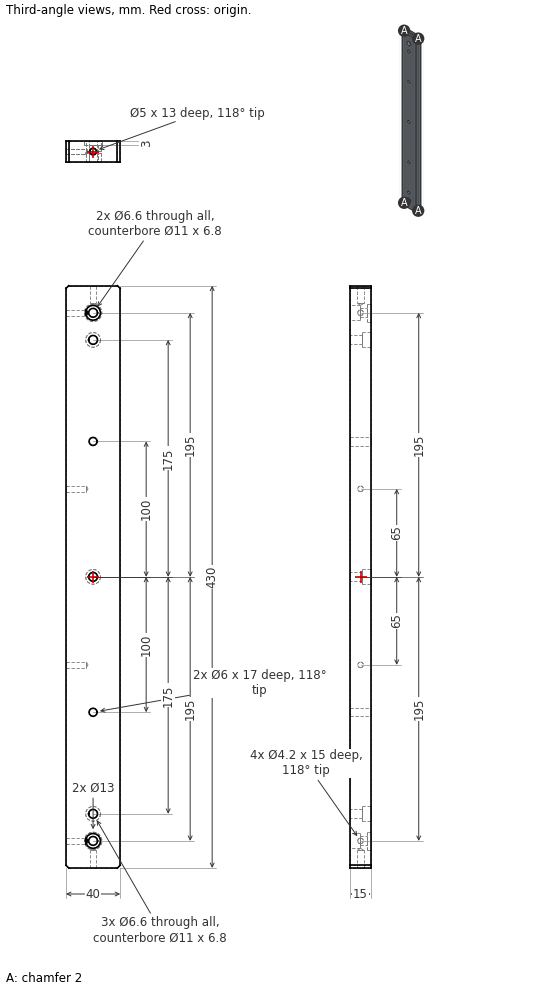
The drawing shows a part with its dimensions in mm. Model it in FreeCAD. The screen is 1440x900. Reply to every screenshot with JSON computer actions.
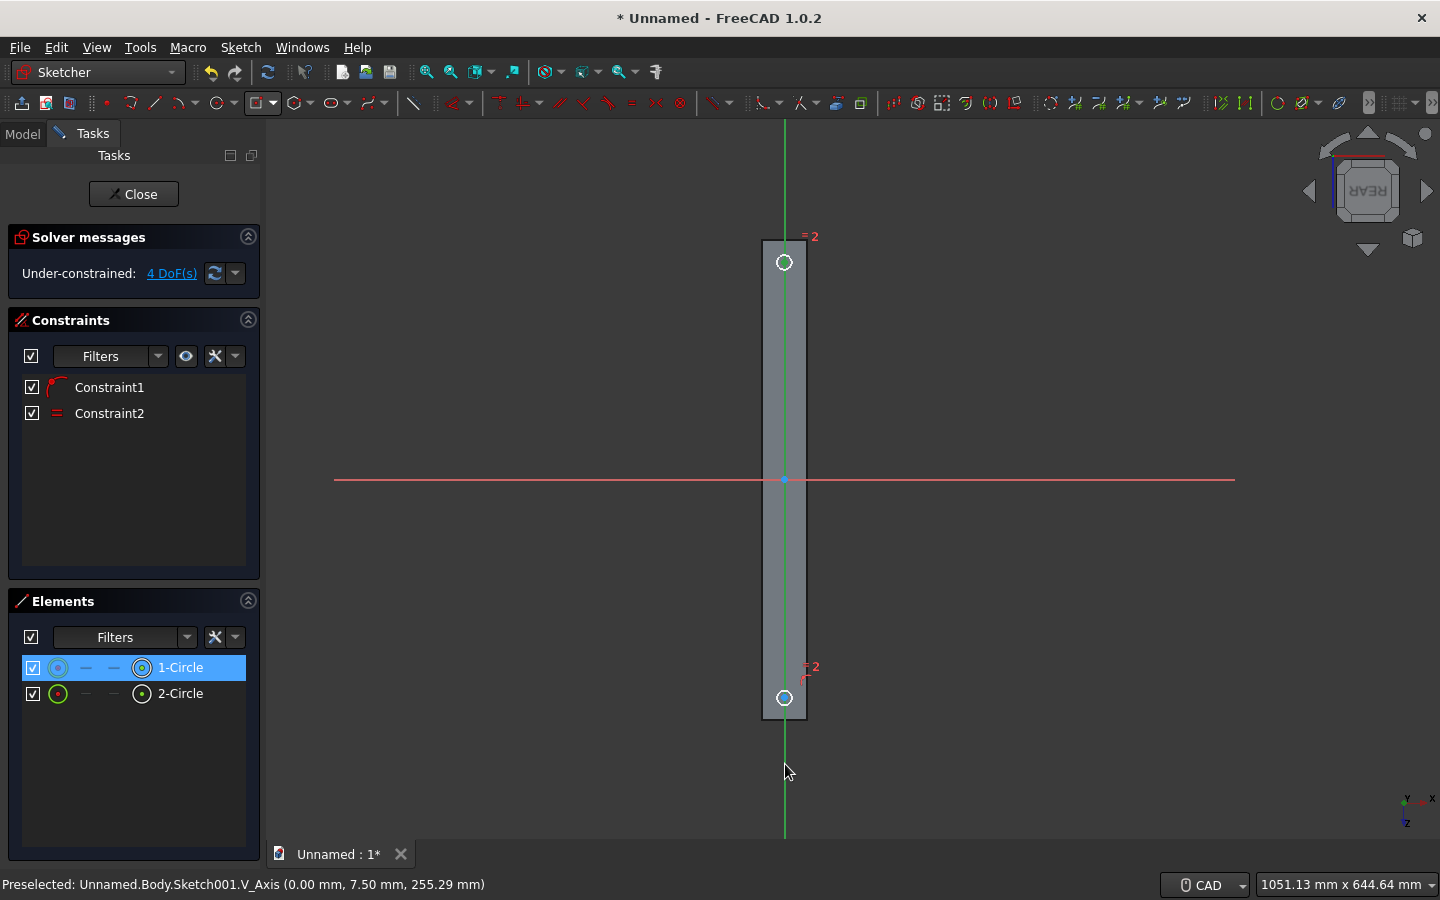
{"action": "left_click", "coordinate": [500, 104]}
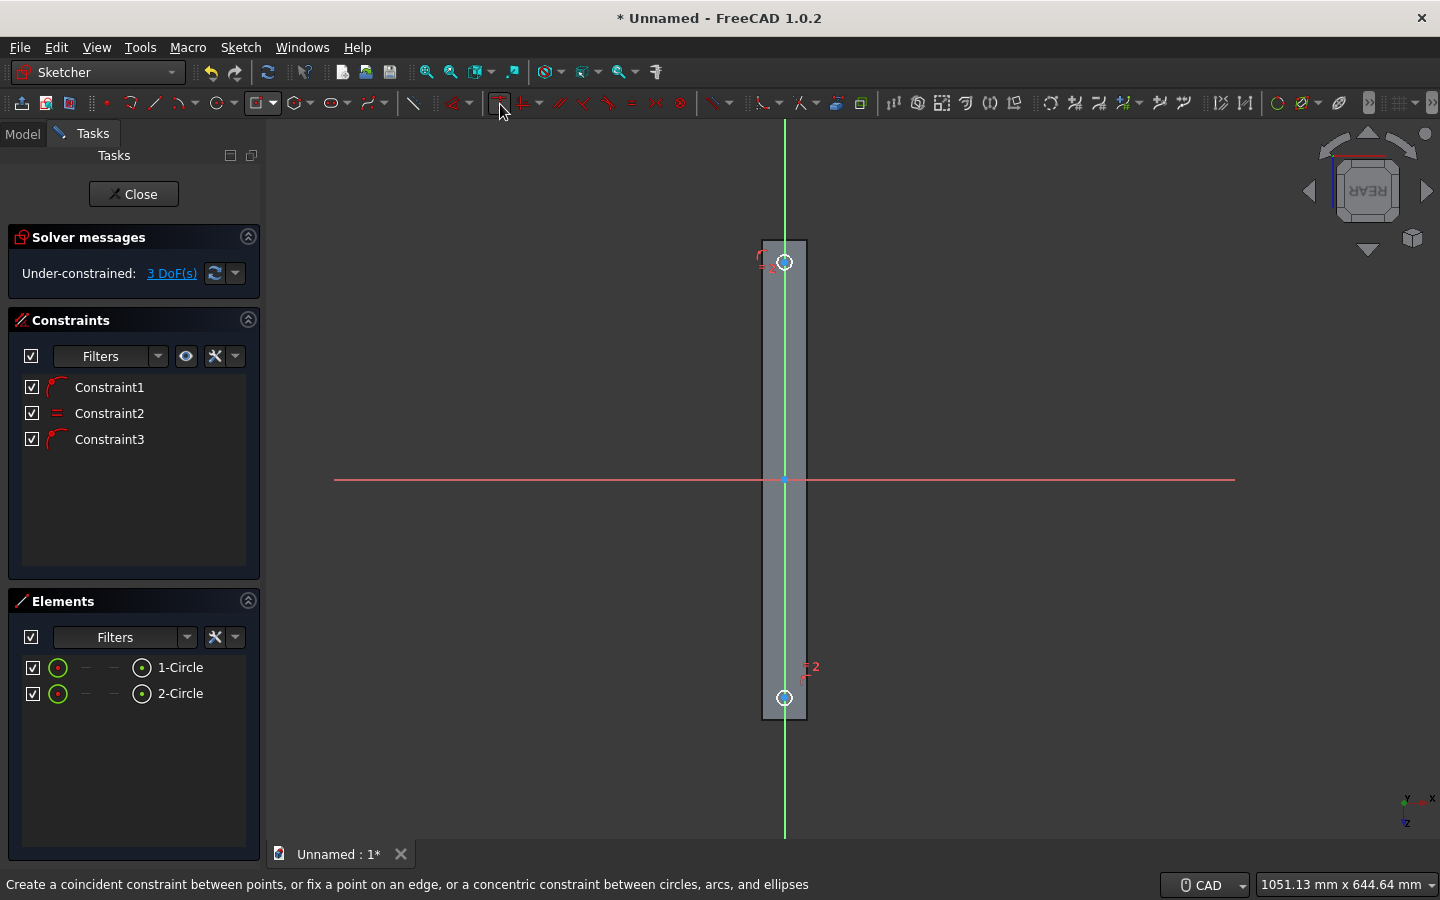
{"action": "key", "text": "d"}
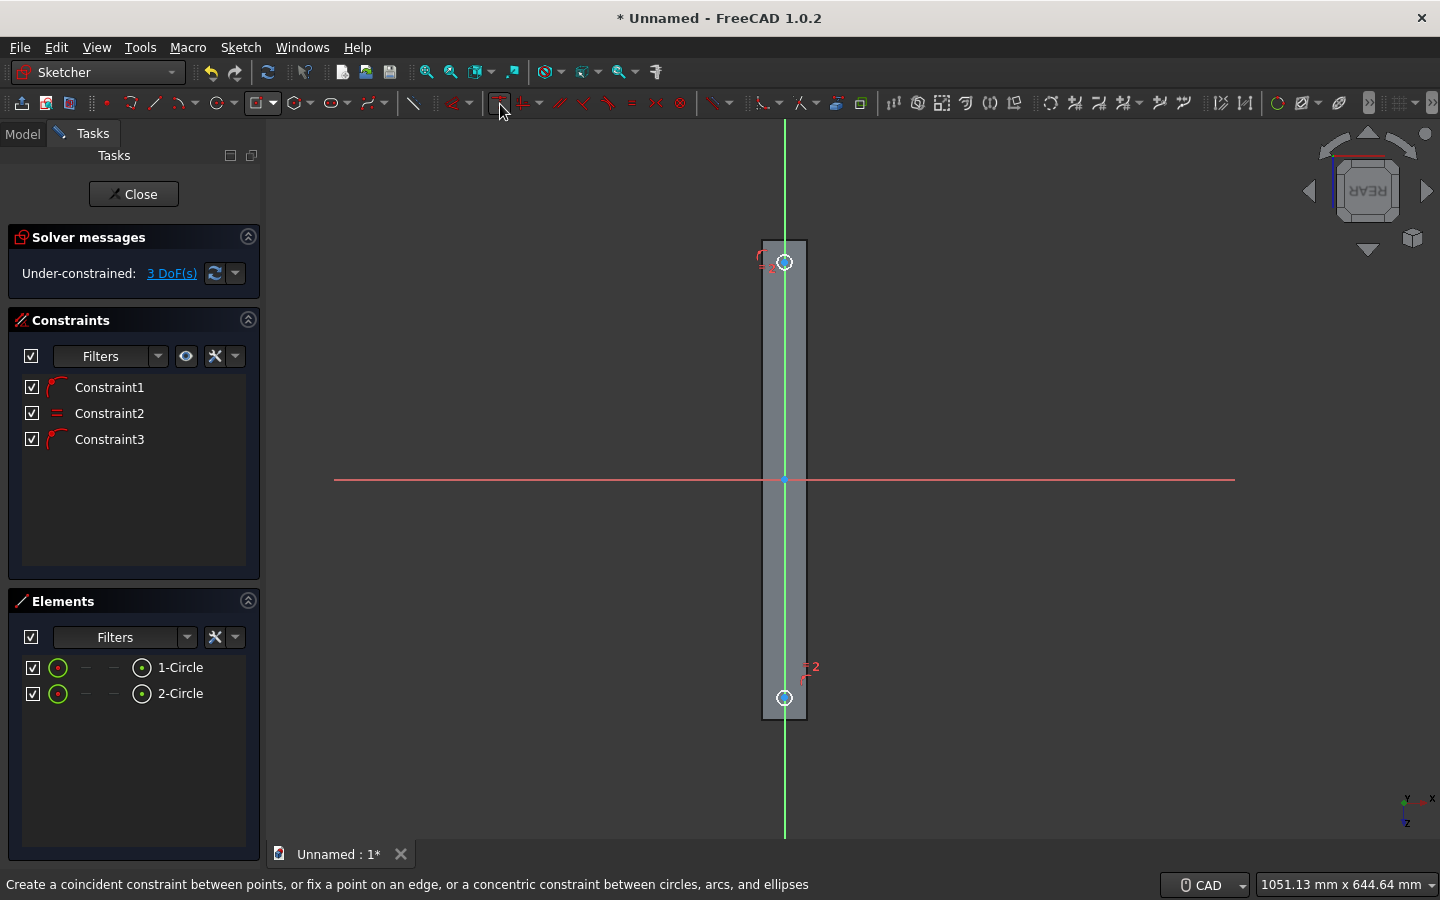
{"action": "scroll", "coordinate": [785, 255], "scroll_direction": "up", "scroll_amount": 6}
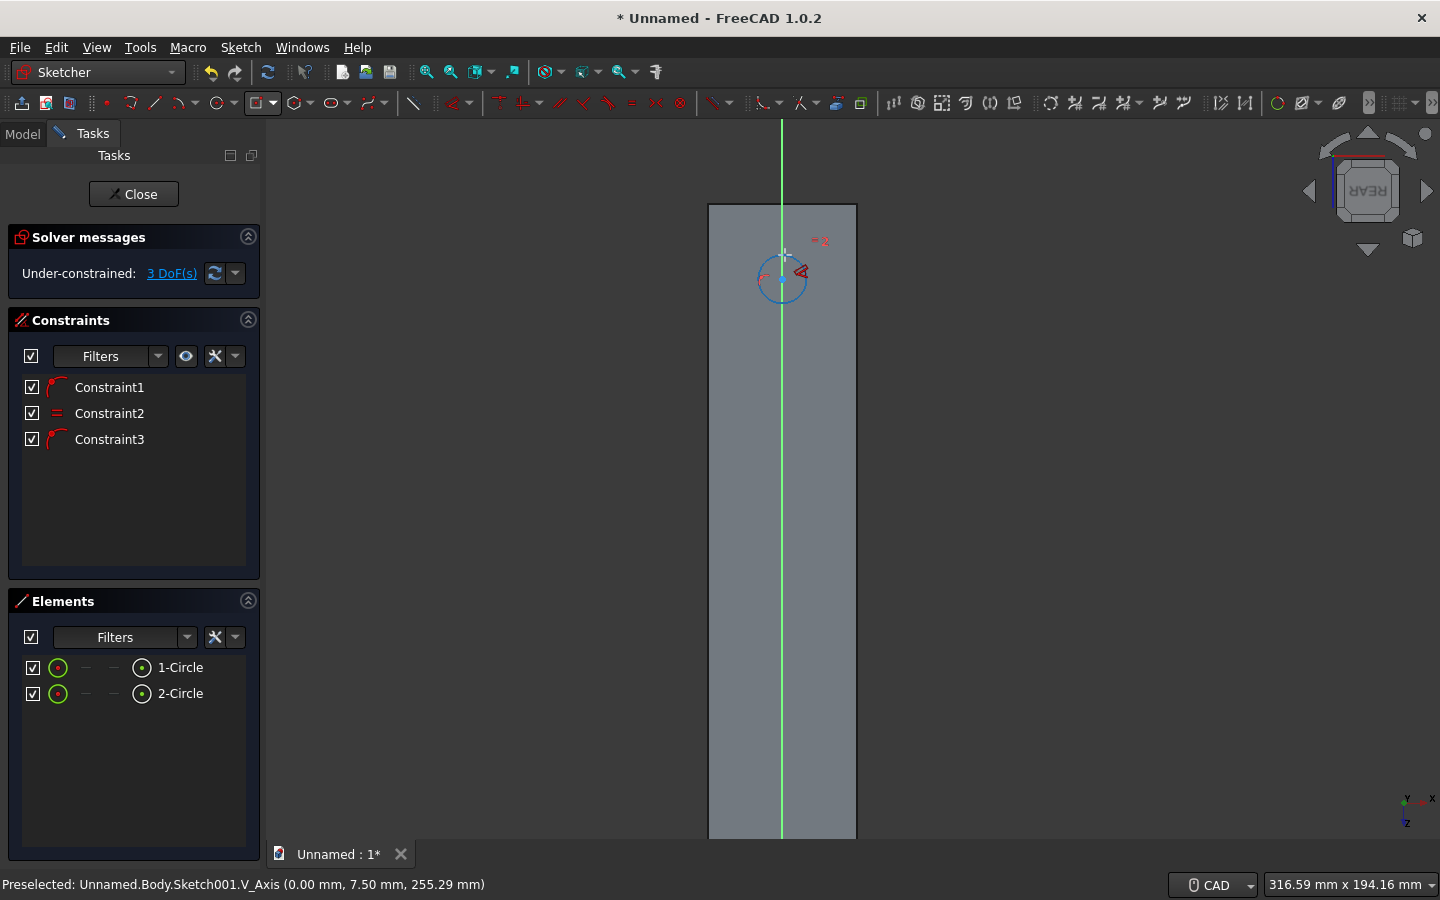
{"action": "left_click", "coordinate": [783, 255]}
{"action": "left_click", "coordinate": [811, 231]}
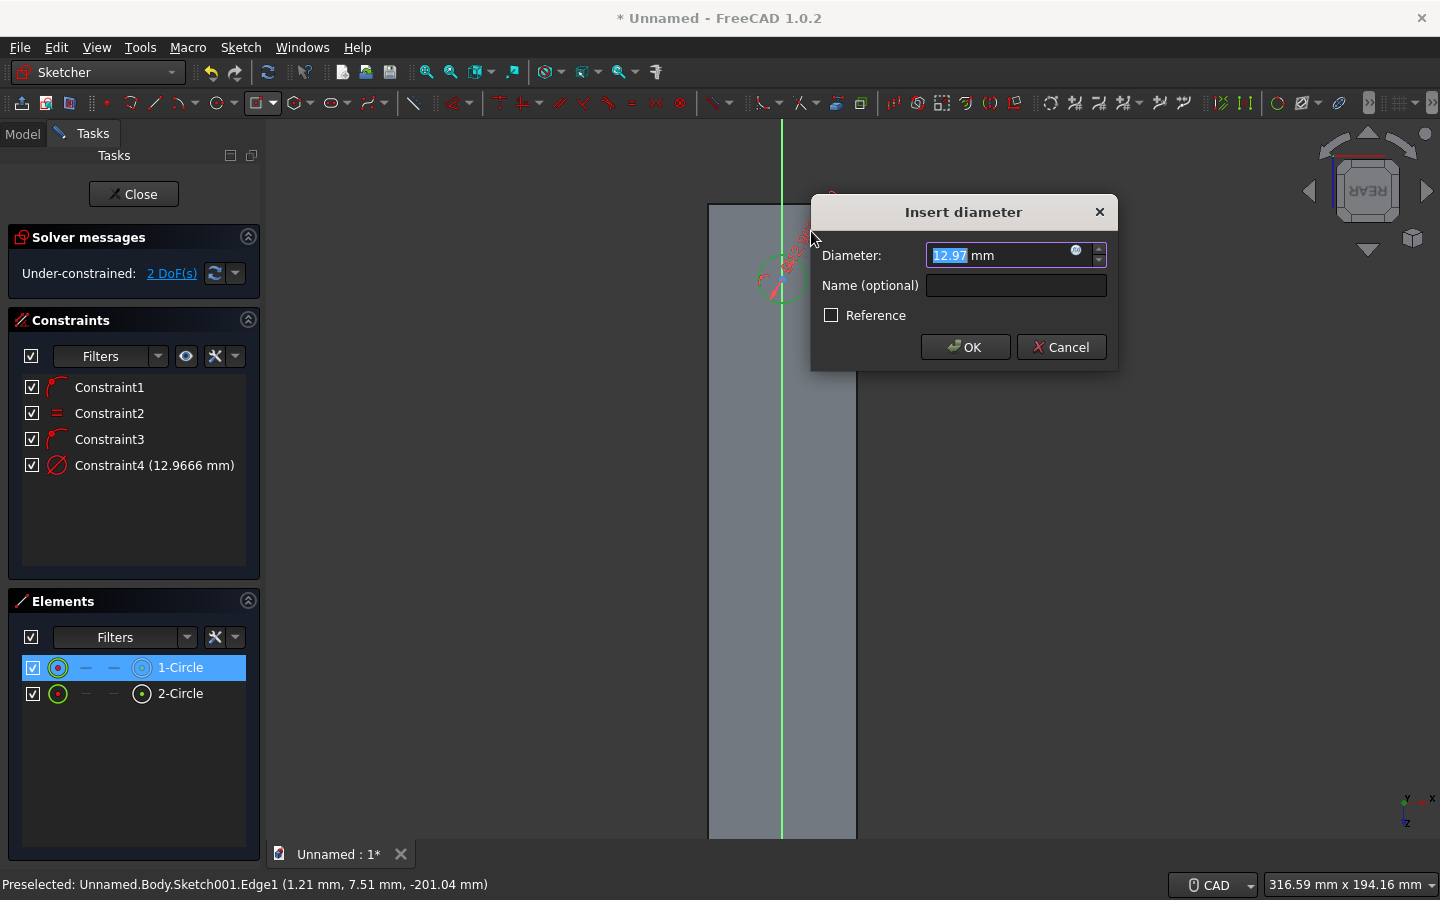
{"action": "type", "text": "13"}
{"action": "key", "text": "Return"}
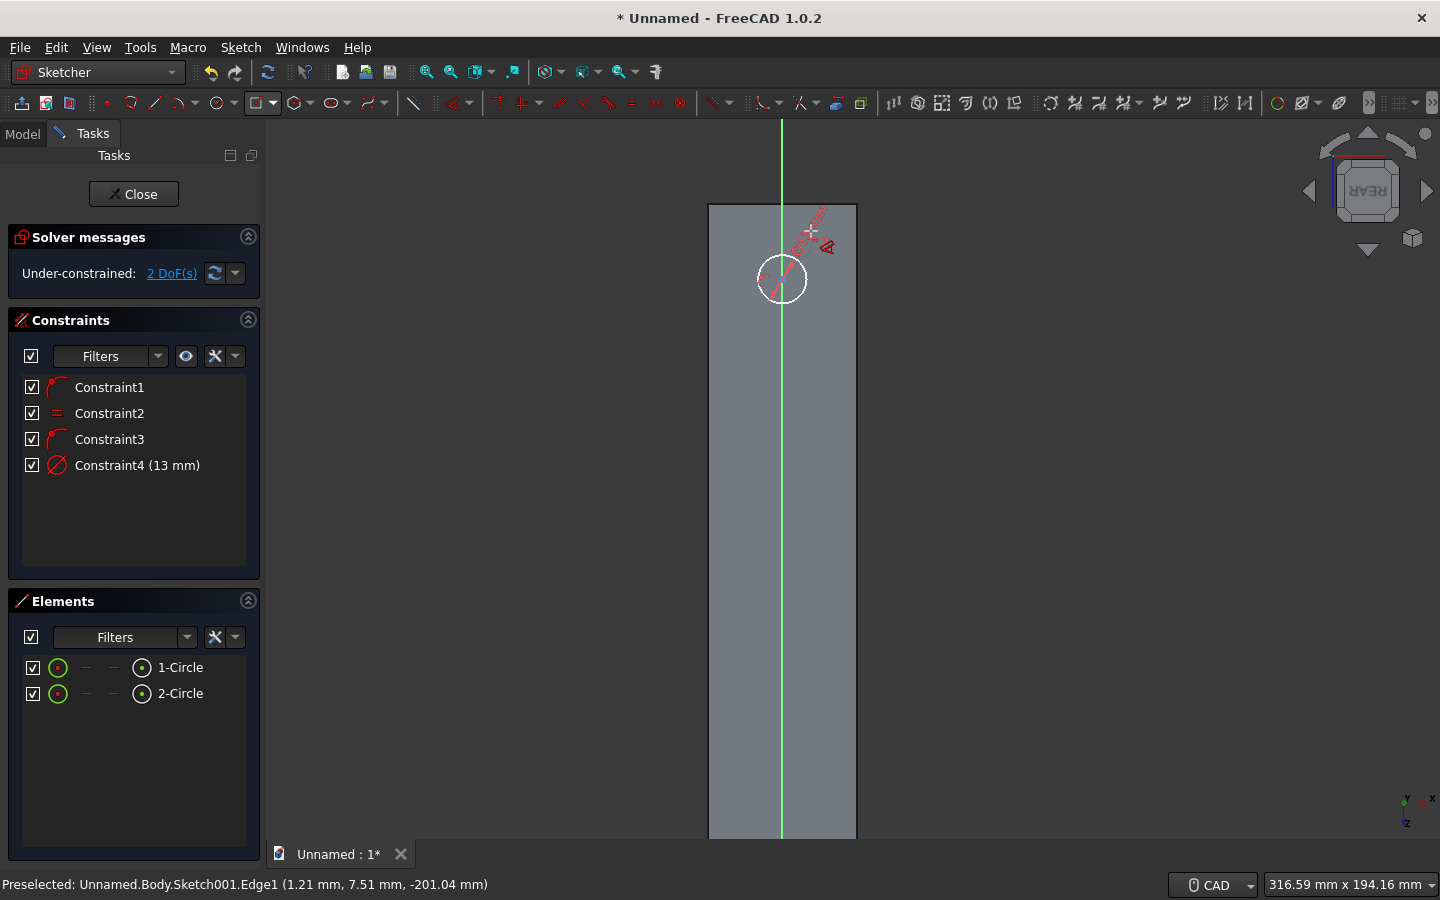
{"action": "left_click", "coordinate": [782, 279]}
{"action": "left_click", "coordinate": [816, 545]}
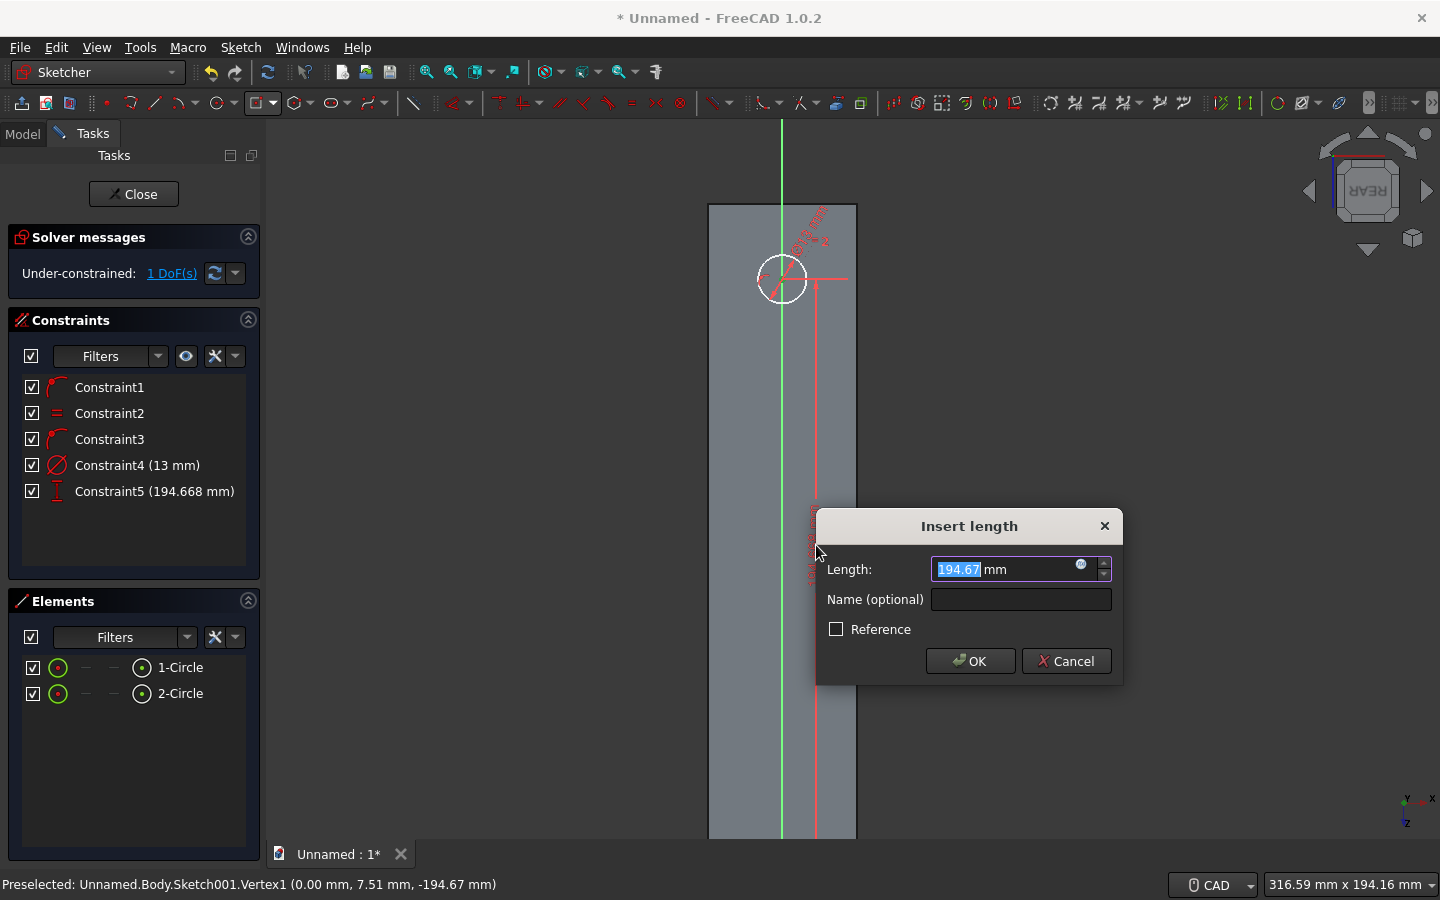
{"action": "type", "text": "195"}
{"action": "key", "text": "Return"}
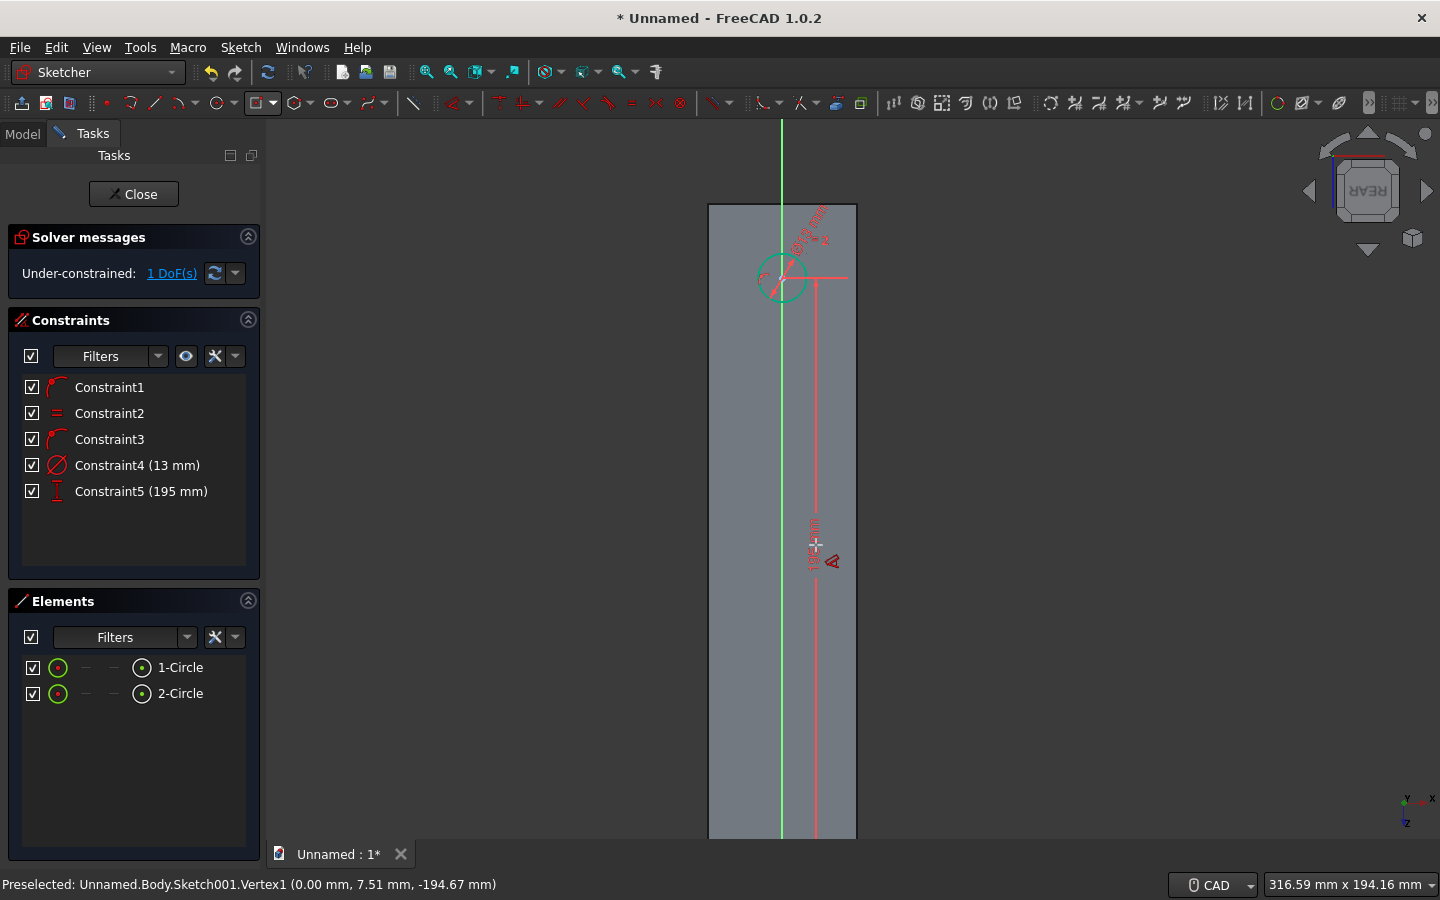
{"action": "scroll", "coordinate": [785, 254], "scroll_direction": "down", "scroll_amount": 6}